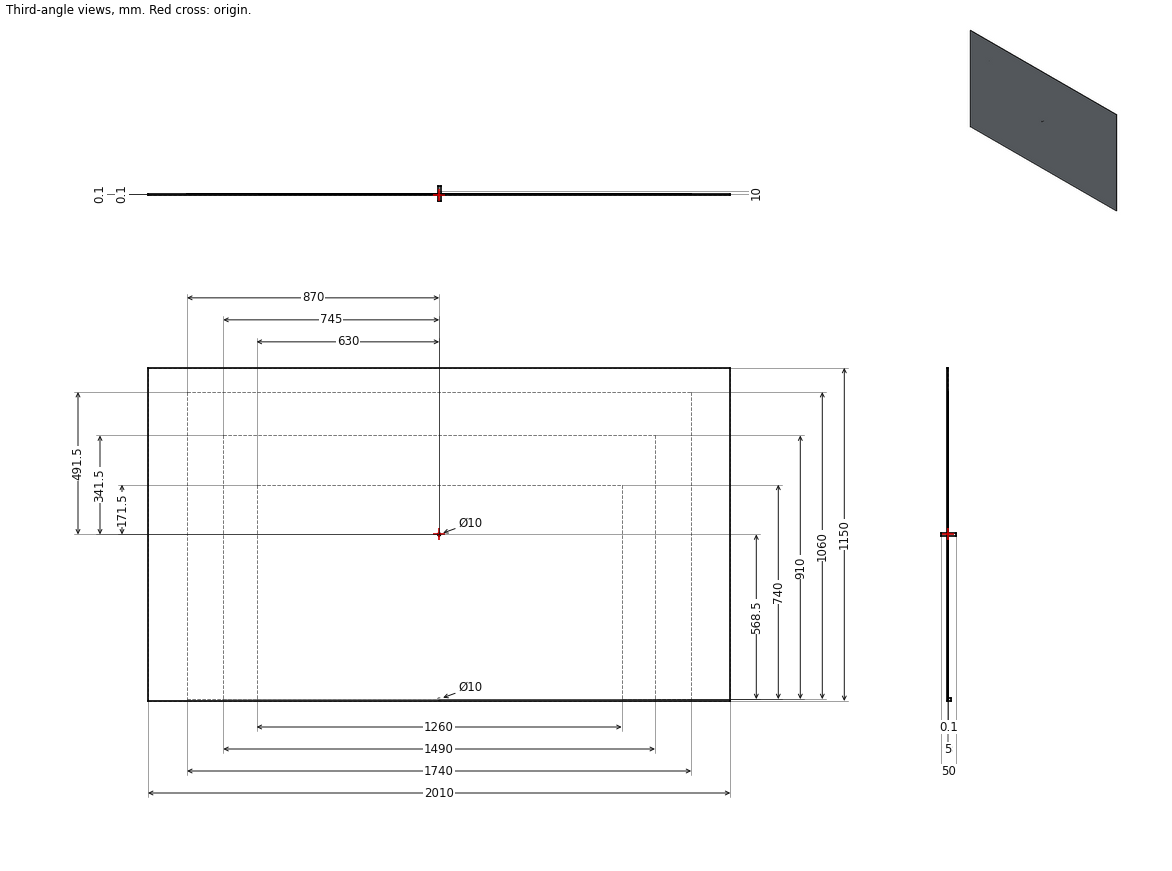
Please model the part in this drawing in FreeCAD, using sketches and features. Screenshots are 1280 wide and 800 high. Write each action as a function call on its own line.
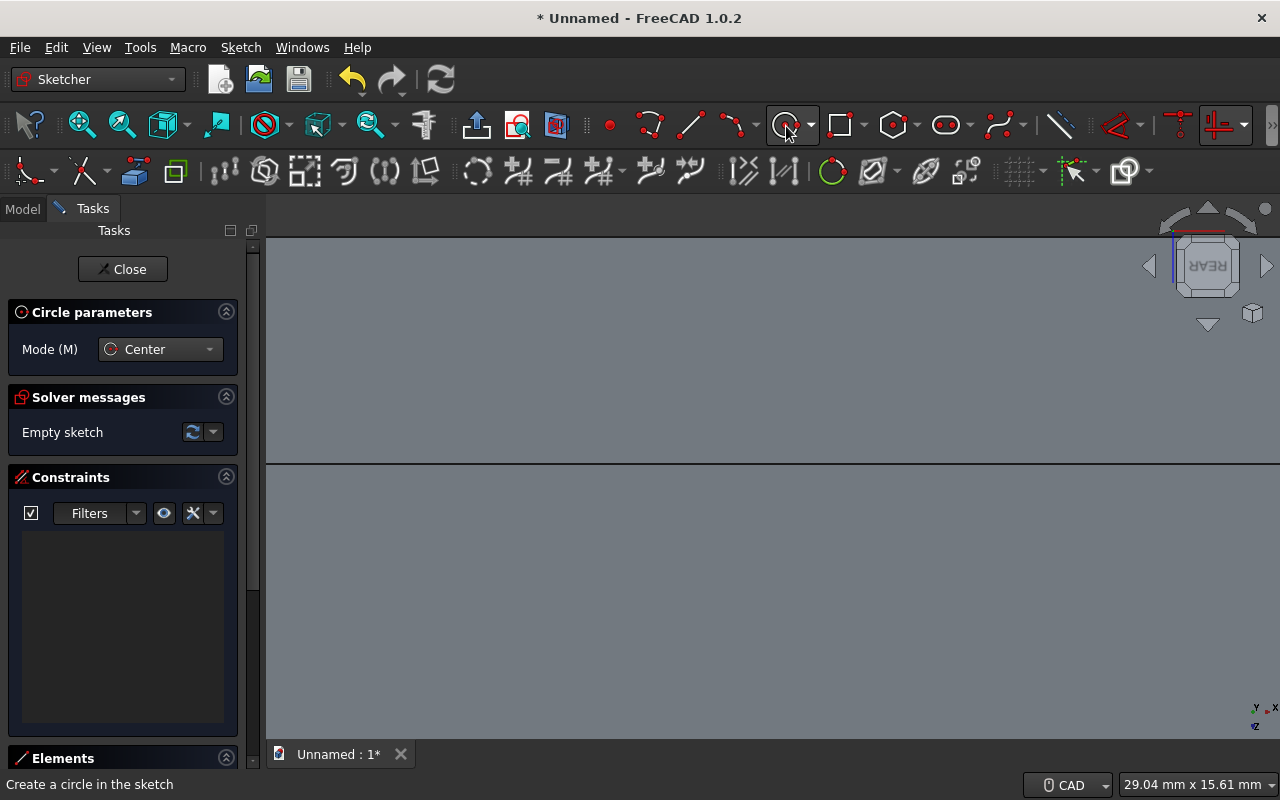
click(704, 464)
move(827, 341)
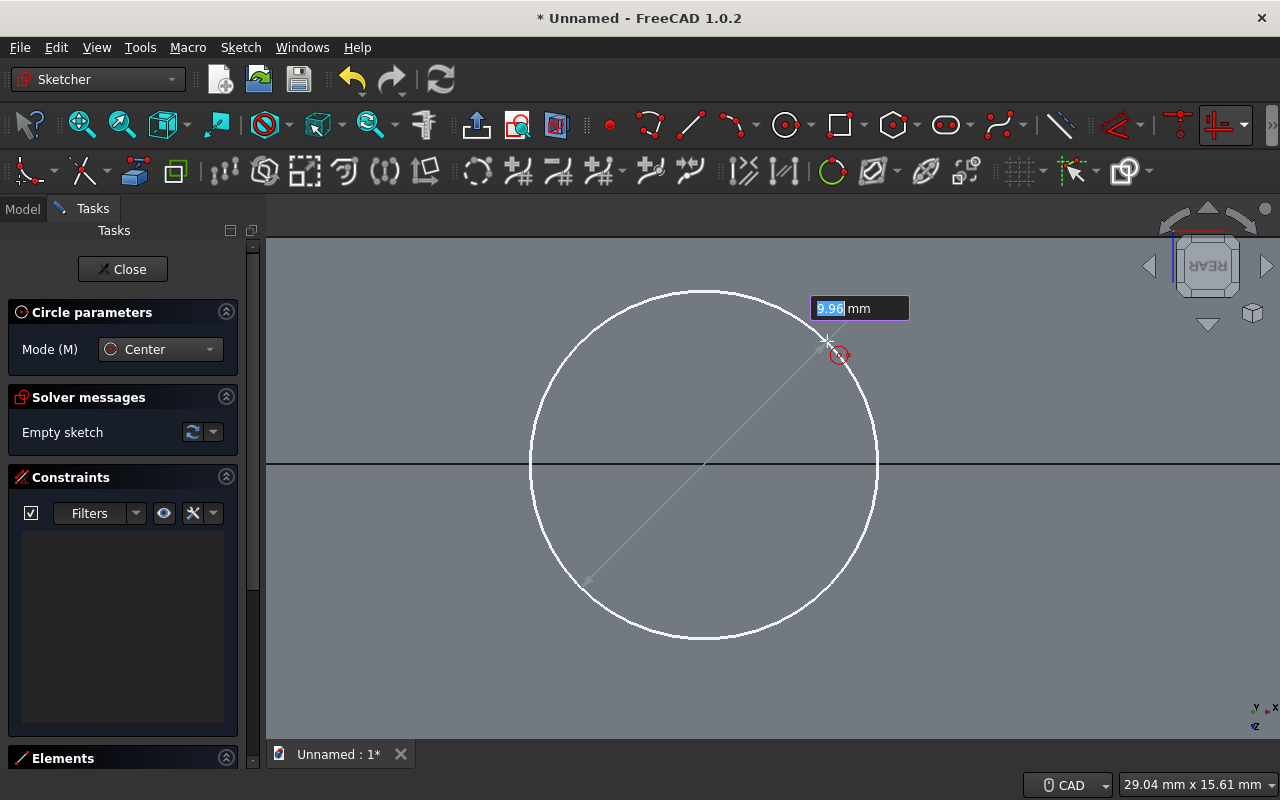
text(10)
key(Return)
key(Escape)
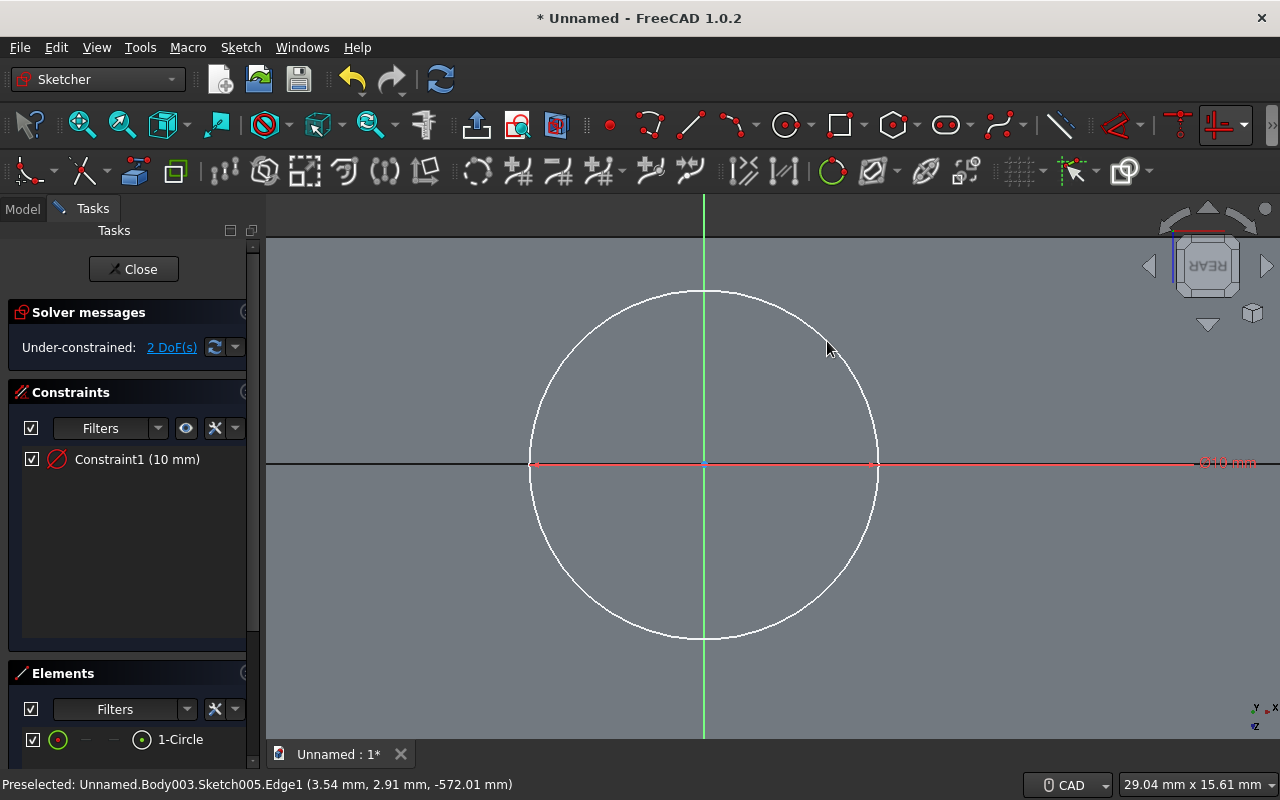
click(704, 465)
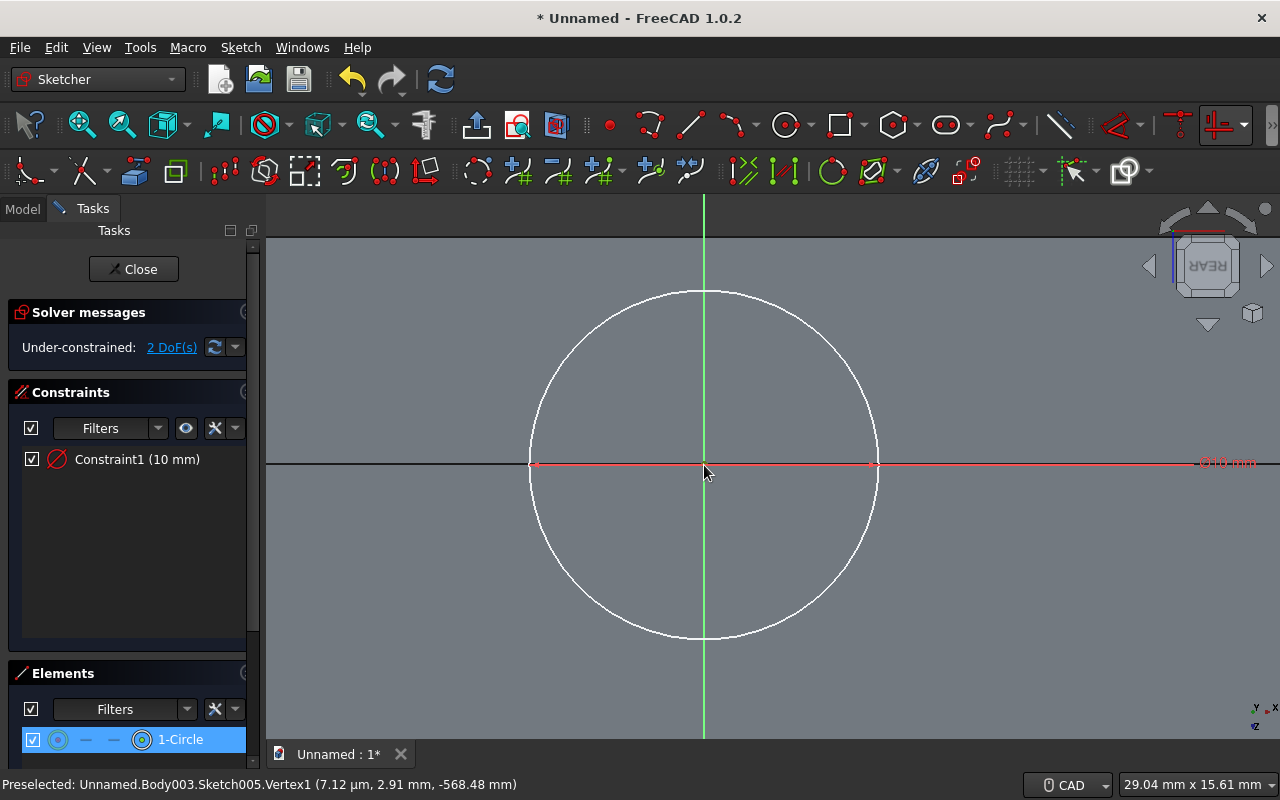
click(704, 676)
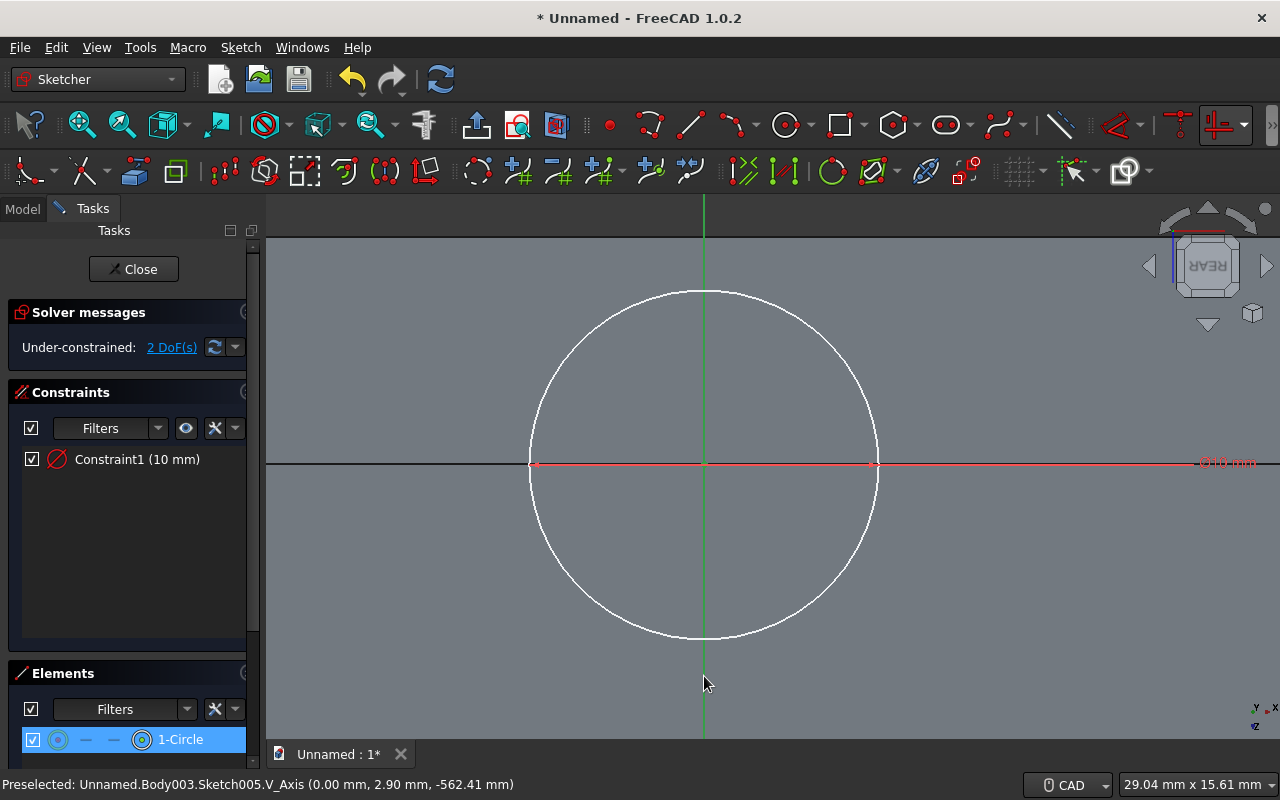
click(1178, 126)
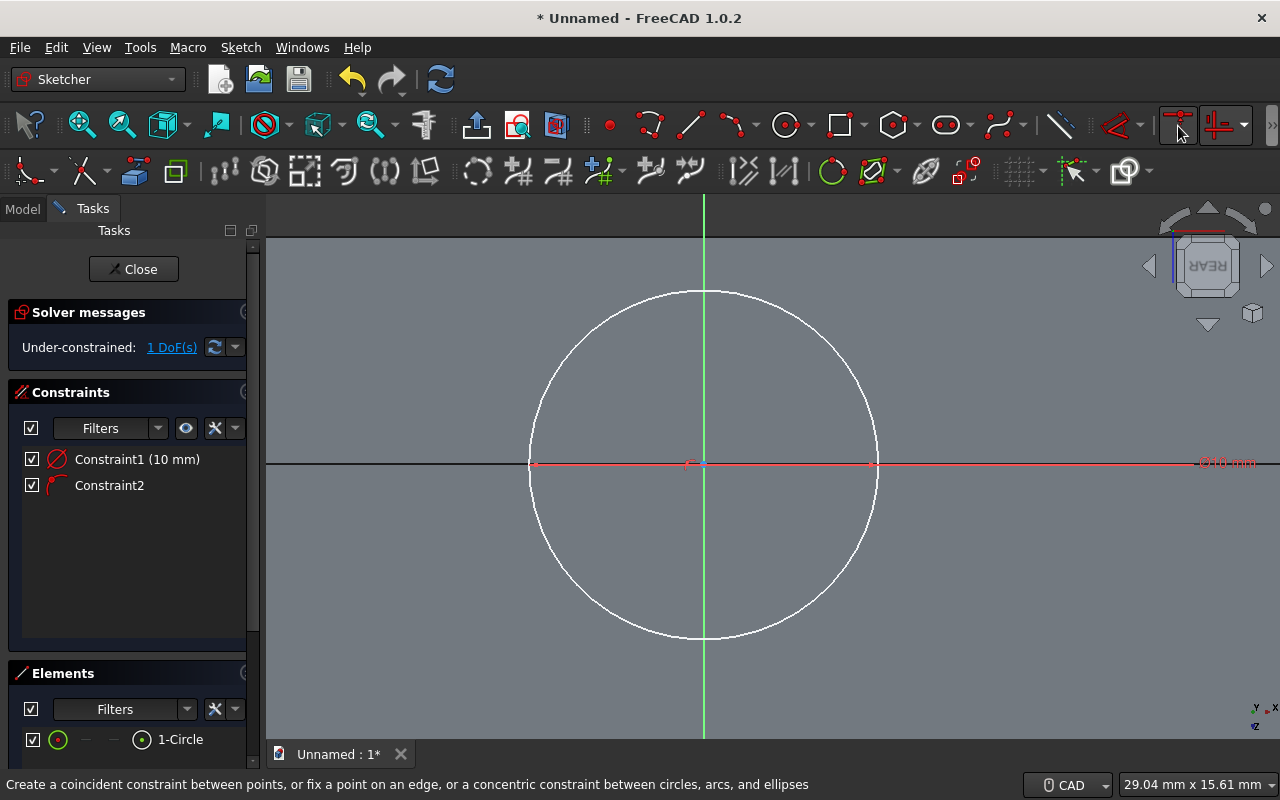
click(1116, 126)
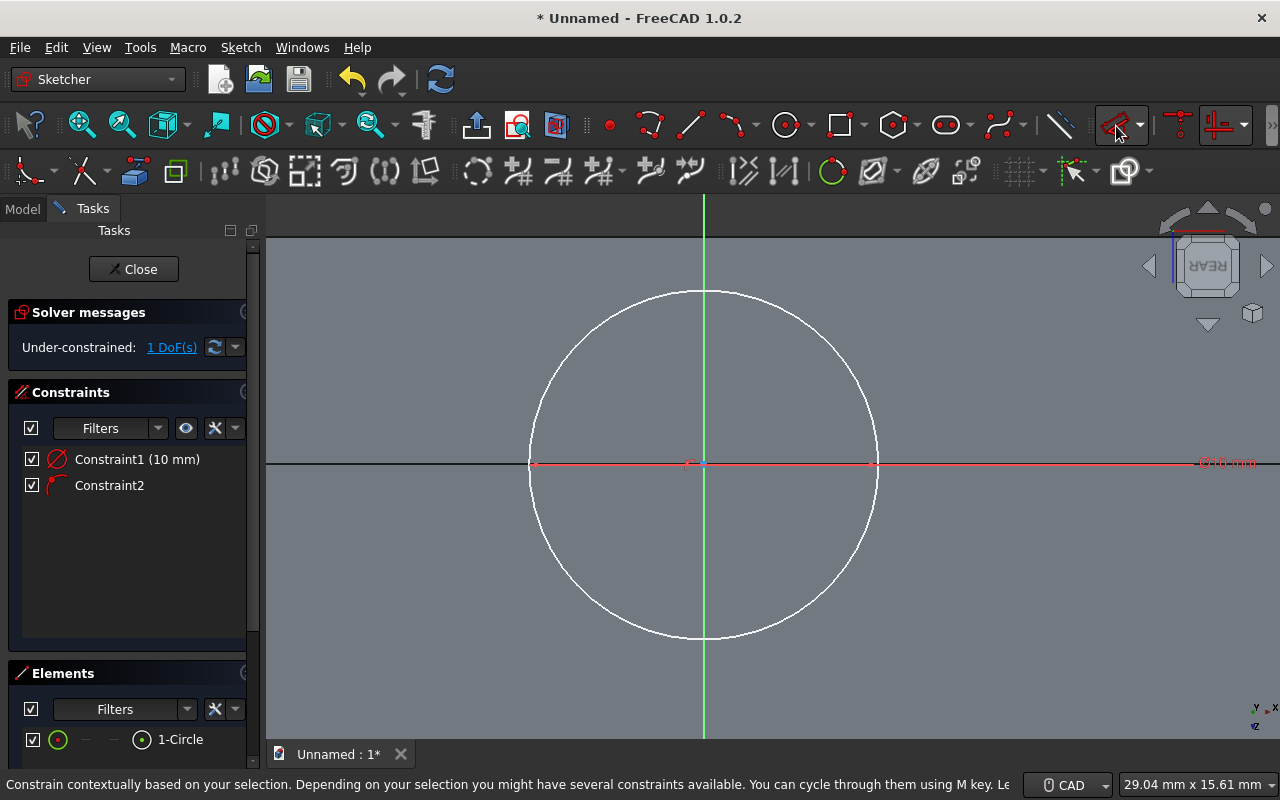
click(704, 465)
click(738, 588)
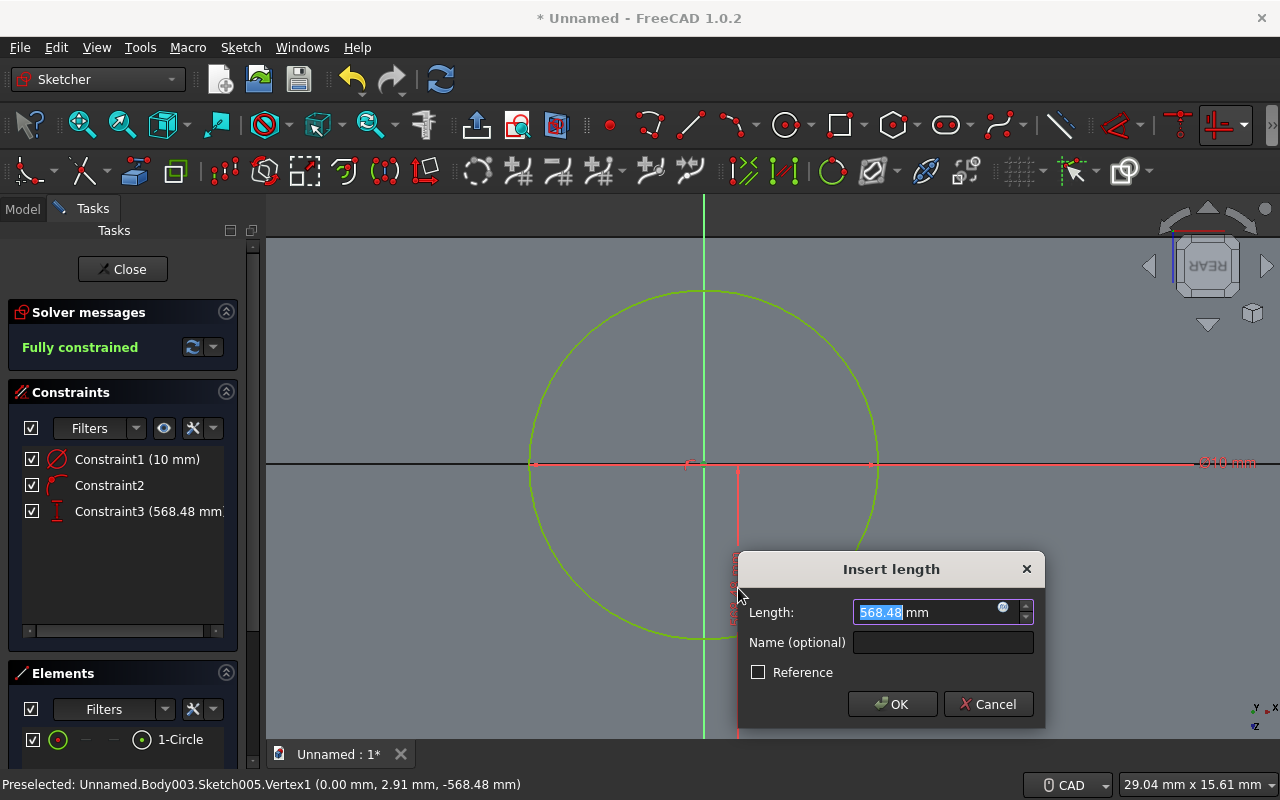
text(568.5)
key(Return)
key(Escape)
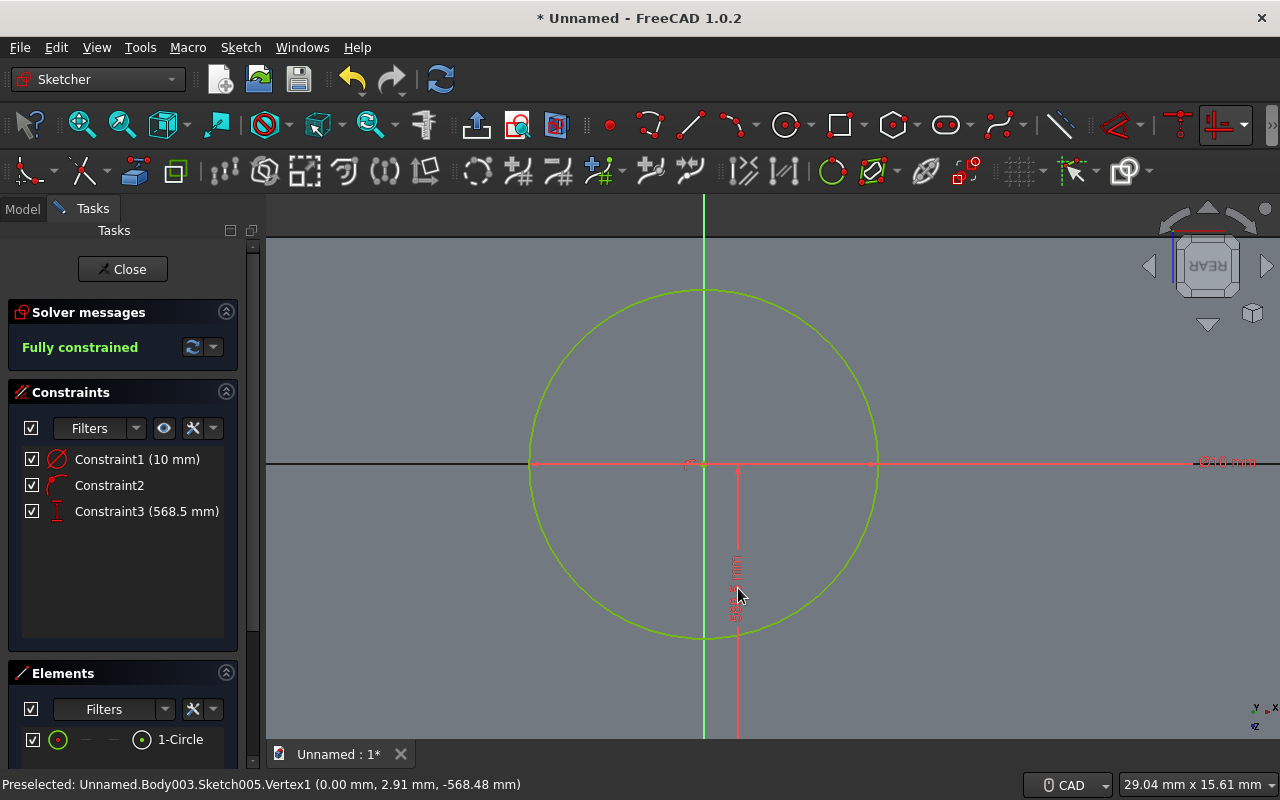
click(123, 269)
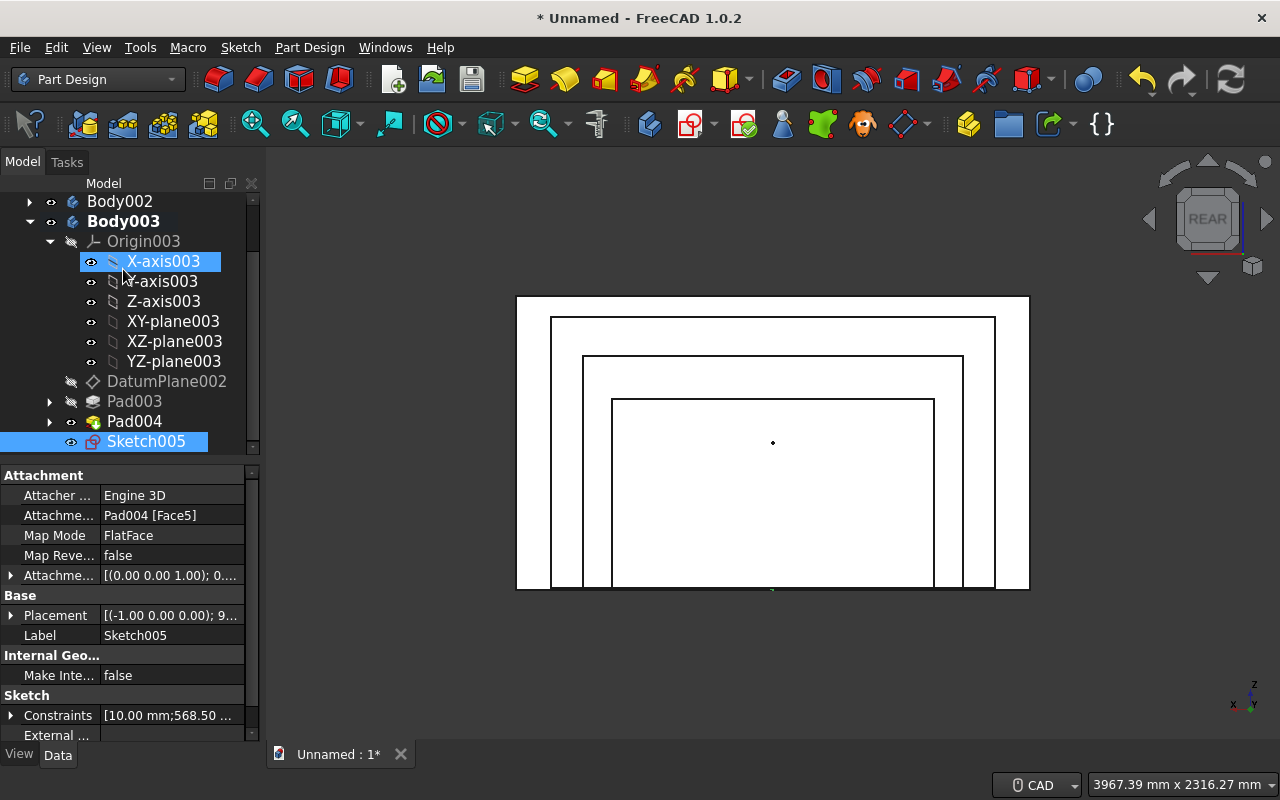
click(526, 80)